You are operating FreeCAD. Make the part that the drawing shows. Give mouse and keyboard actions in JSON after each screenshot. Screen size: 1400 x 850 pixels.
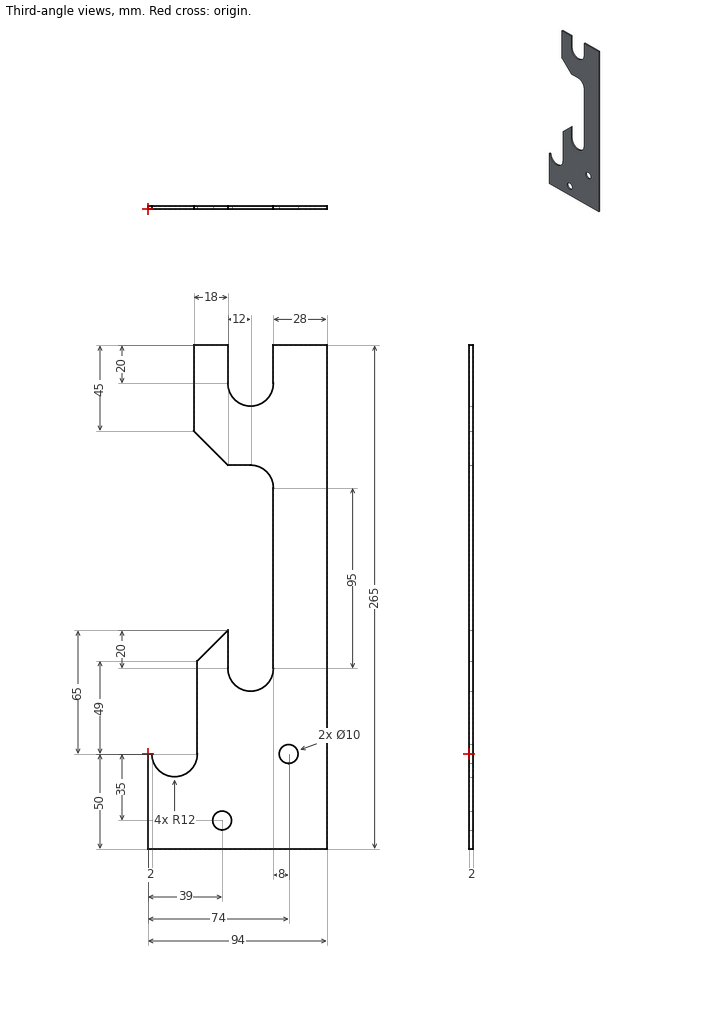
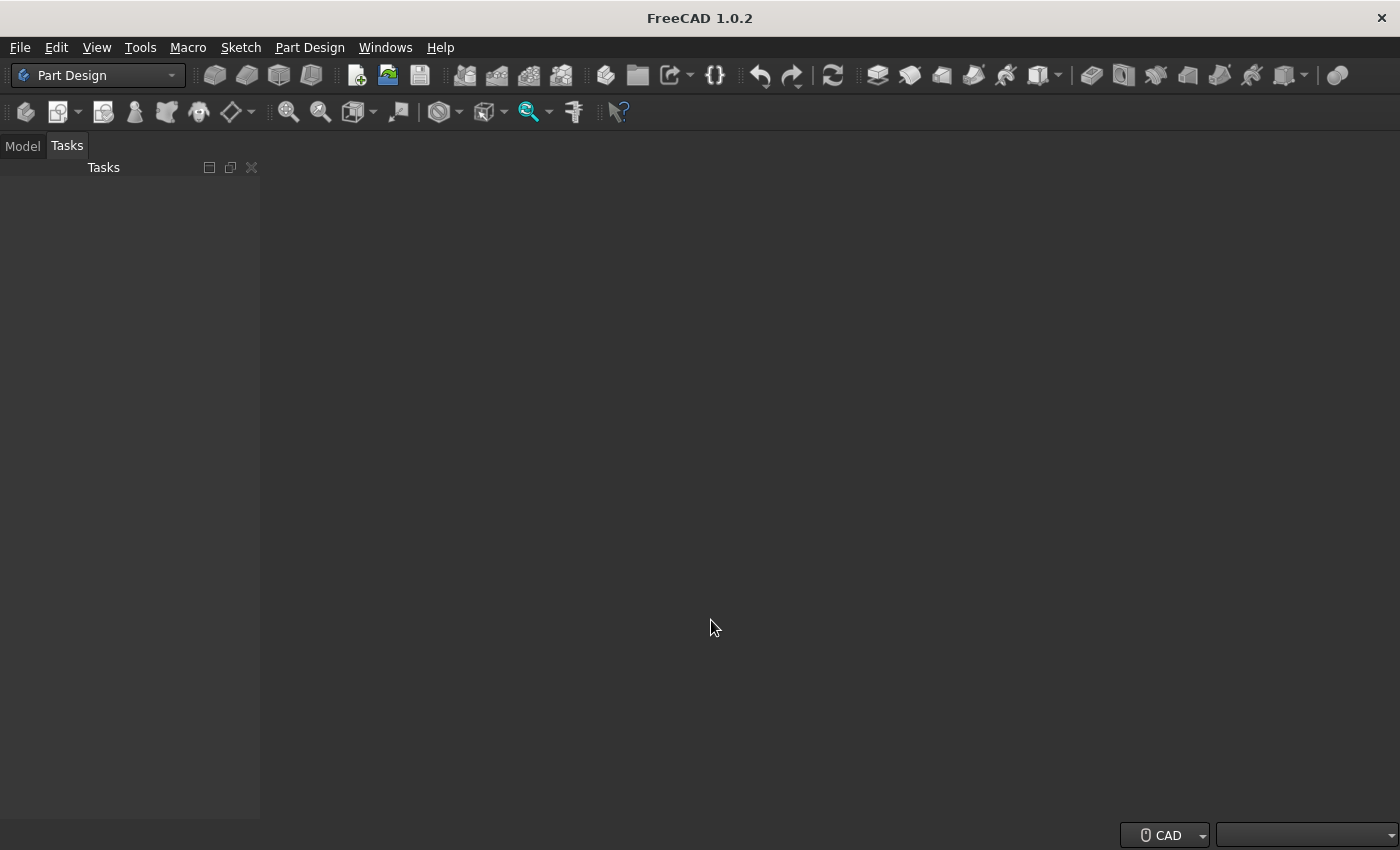
{"action": "key", "text": "ctrl+n"}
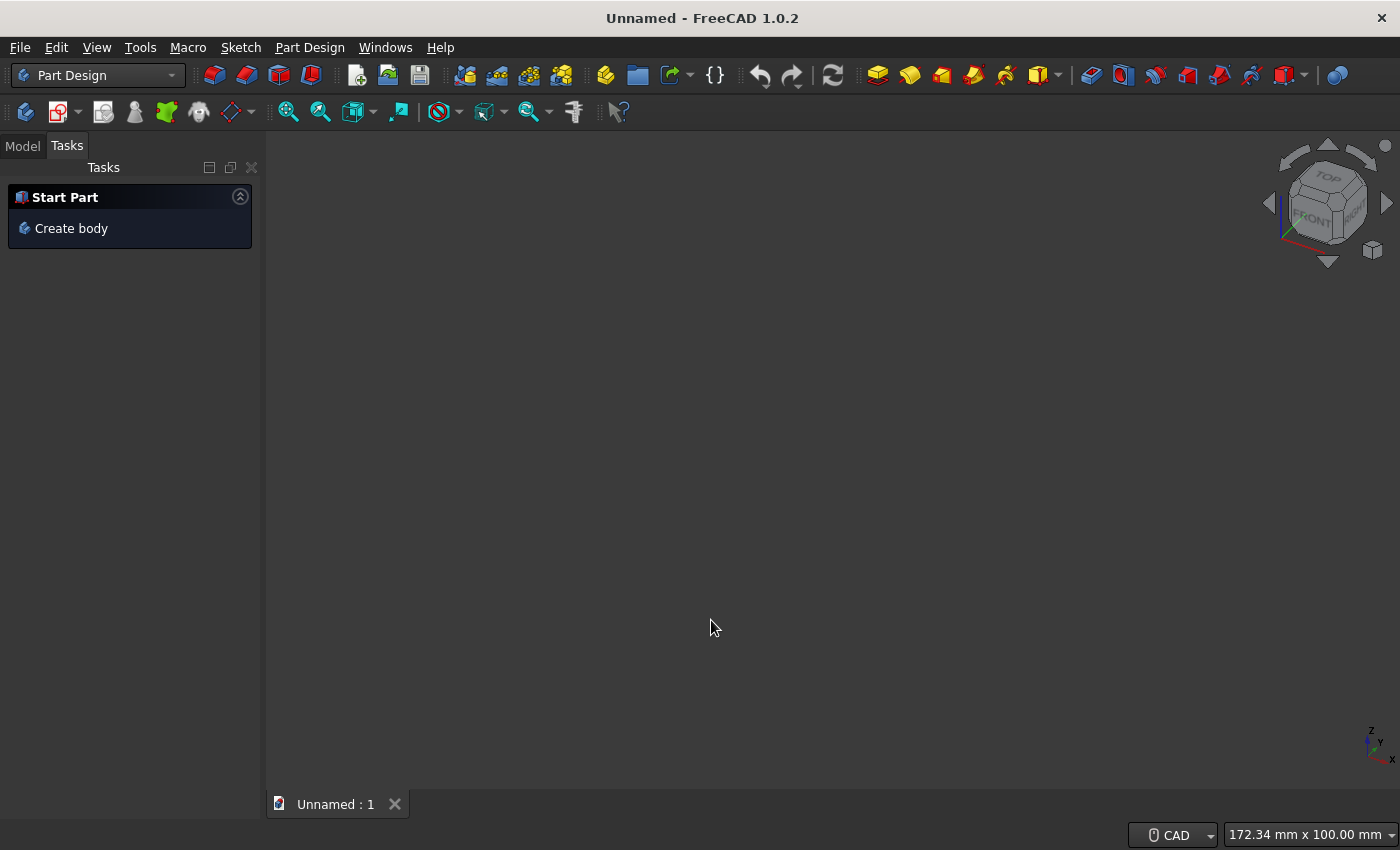
{"action": "left_click", "coordinate": [58, 112]}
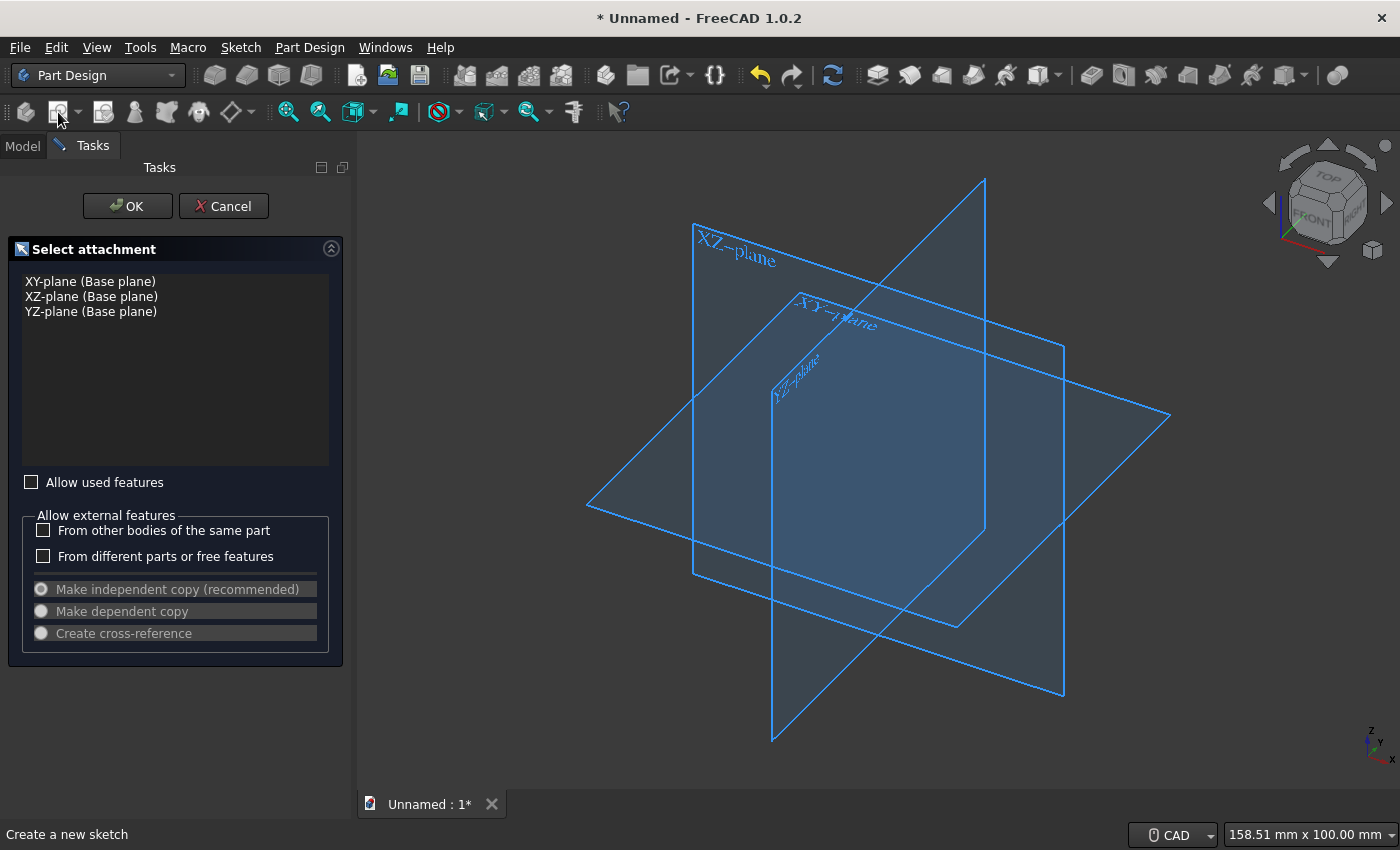
{"action": "left_click", "coordinate": [82, 296]}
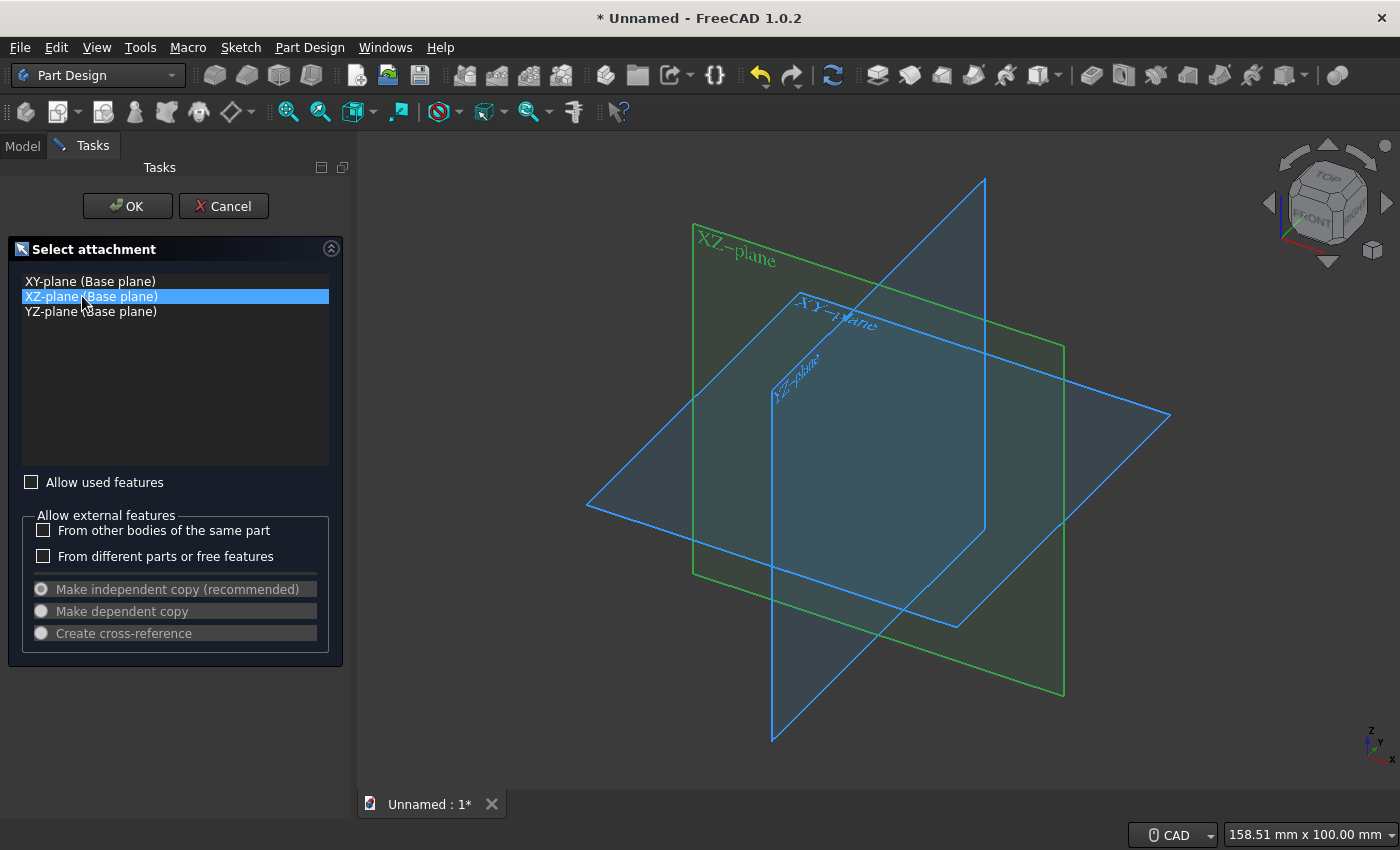
{"action": "left_click", "coordinate": [128, 206]}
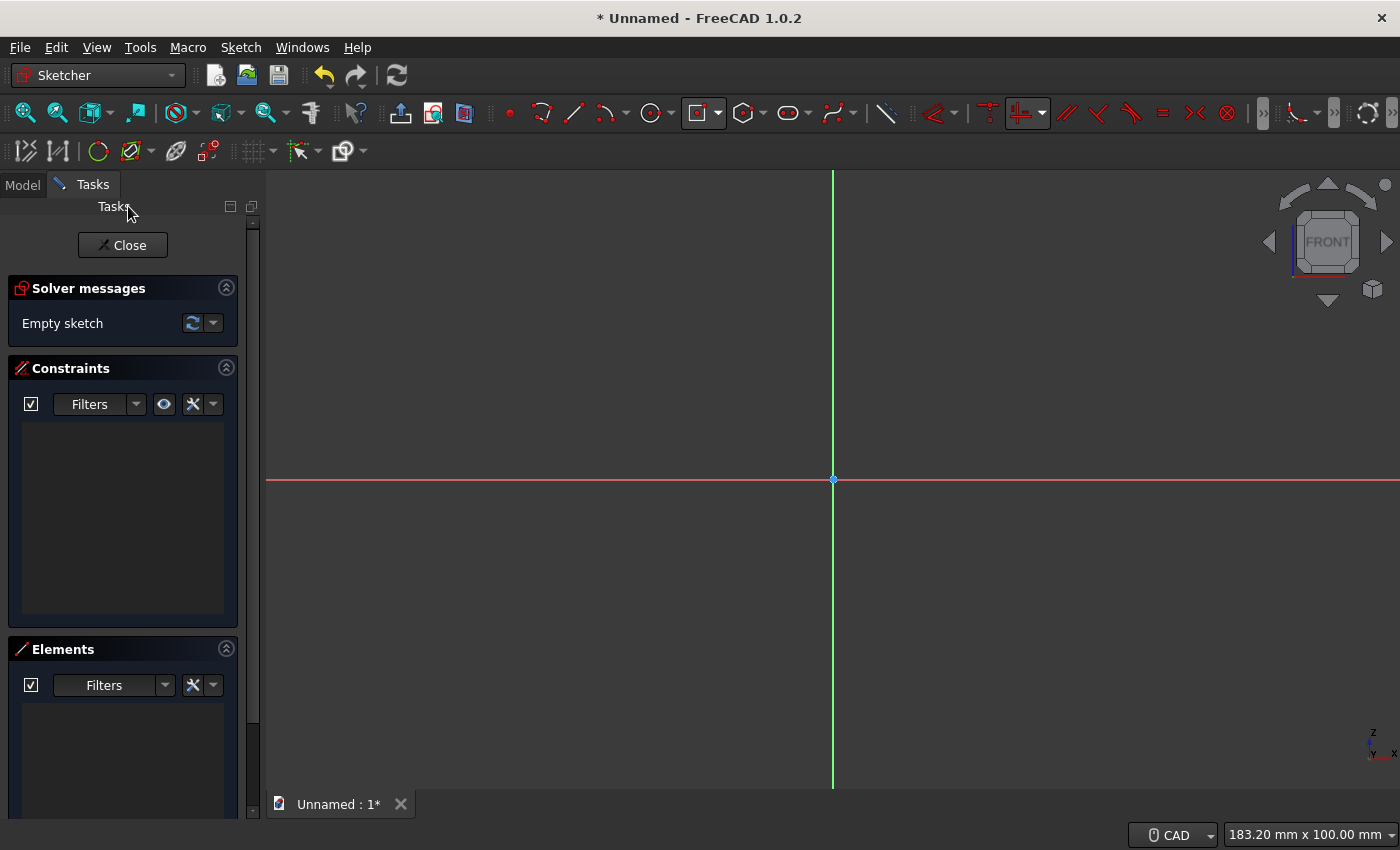
{"action": "scroll", "coordinate": [647, 647], "scroll_direction": "down", "scroll_amount": 7}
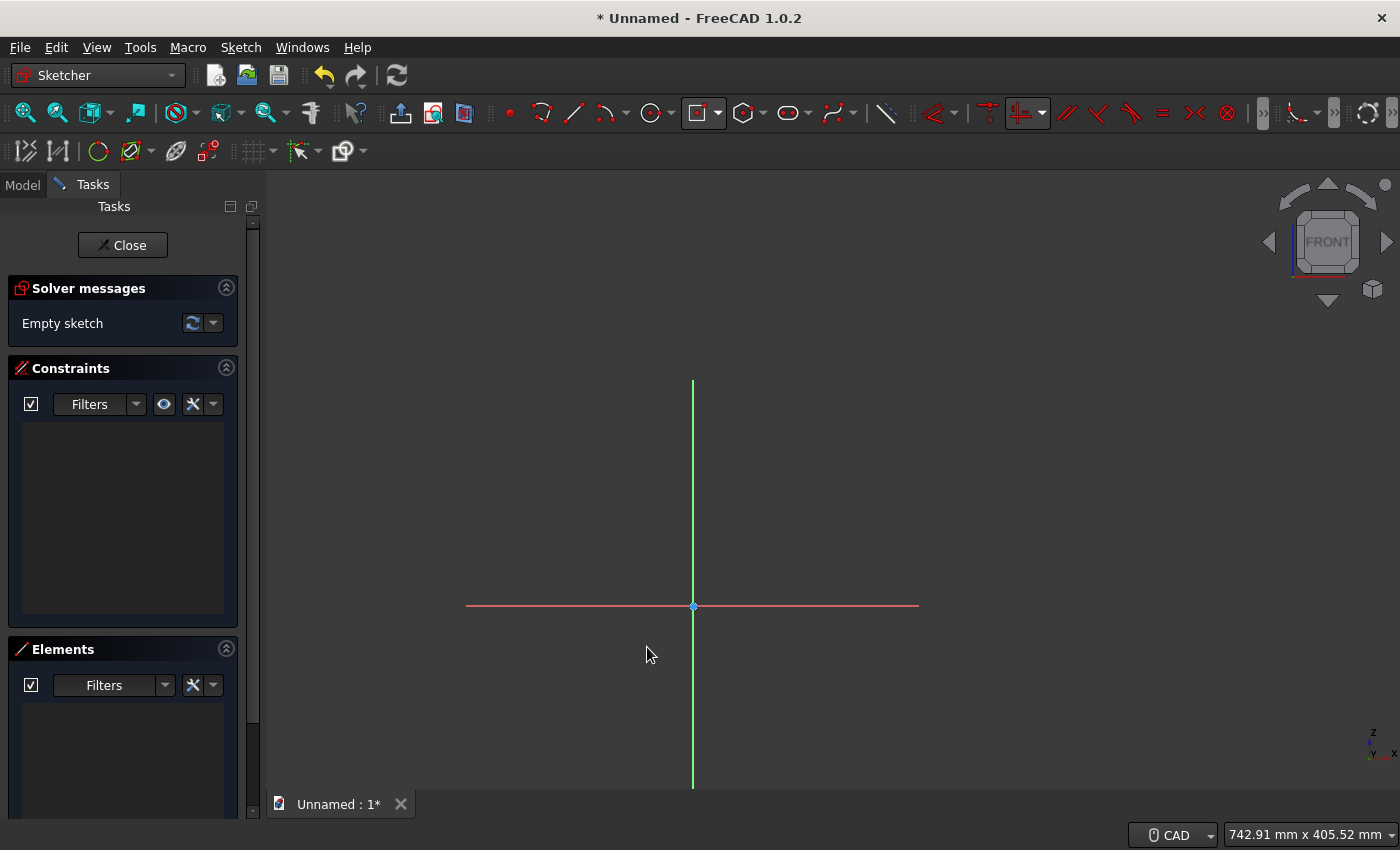
{"action": "key", "text": "g m"}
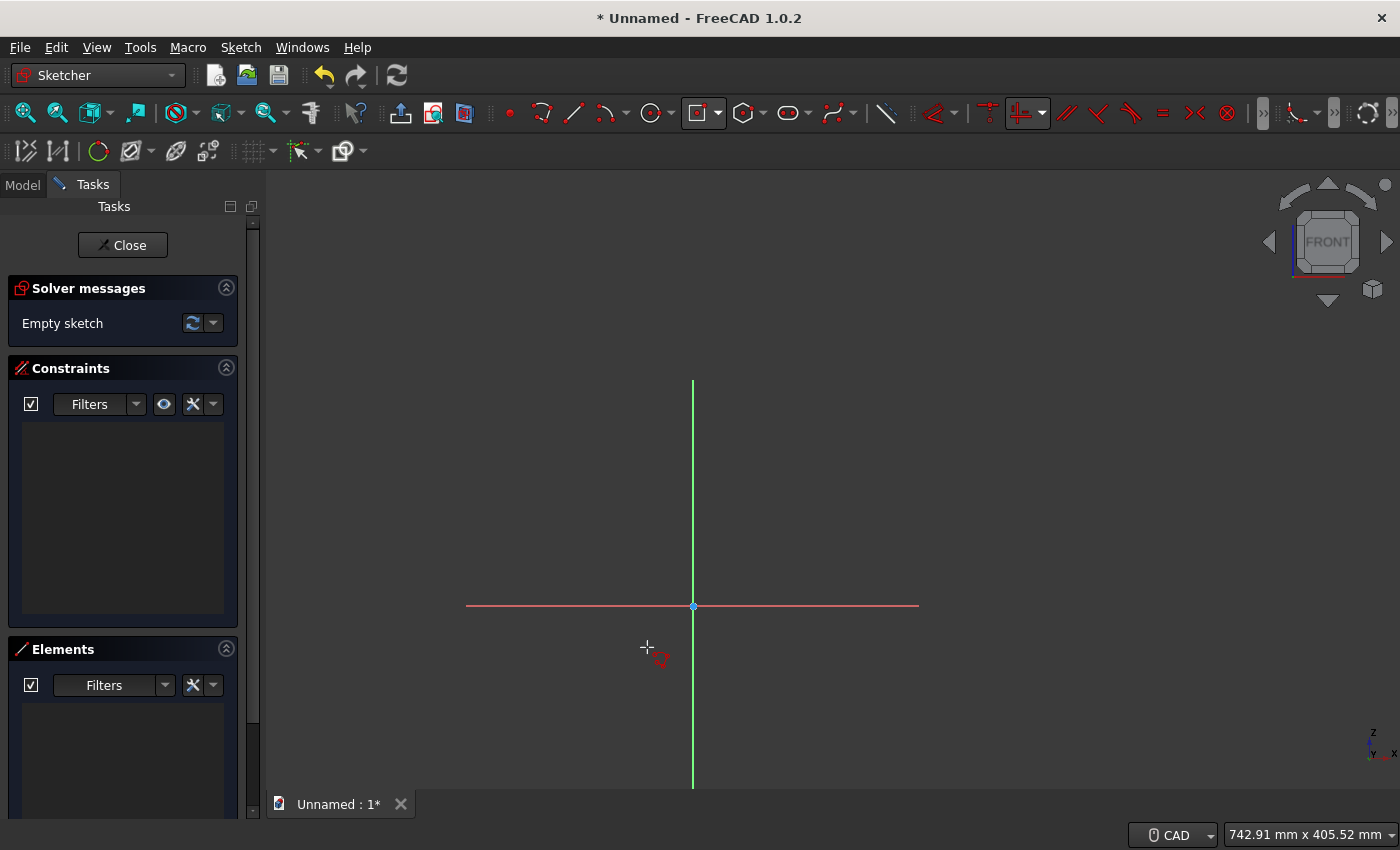
{"action": "left_click", "coordinate": [733, 606]}
{"action": "left_click", "coordinate": [733, 531]}
{"action": "left_click", "coordinate": [757, 507]}
{"action": "left_click", "coordinate": [757, 538]}
{"action": "right_click", "coordinate": [757, 538]}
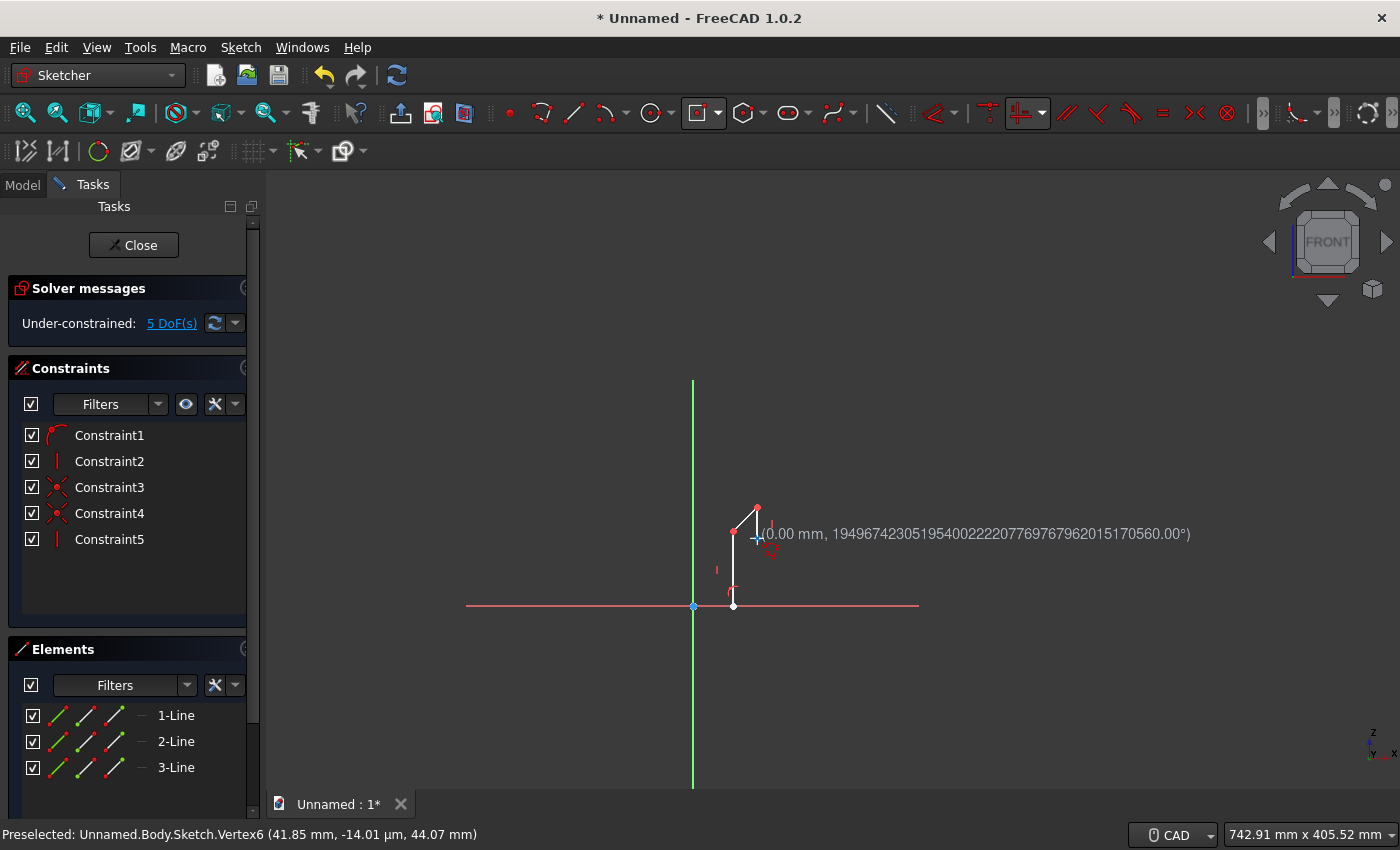
{"action": "key", "text": "g l"}